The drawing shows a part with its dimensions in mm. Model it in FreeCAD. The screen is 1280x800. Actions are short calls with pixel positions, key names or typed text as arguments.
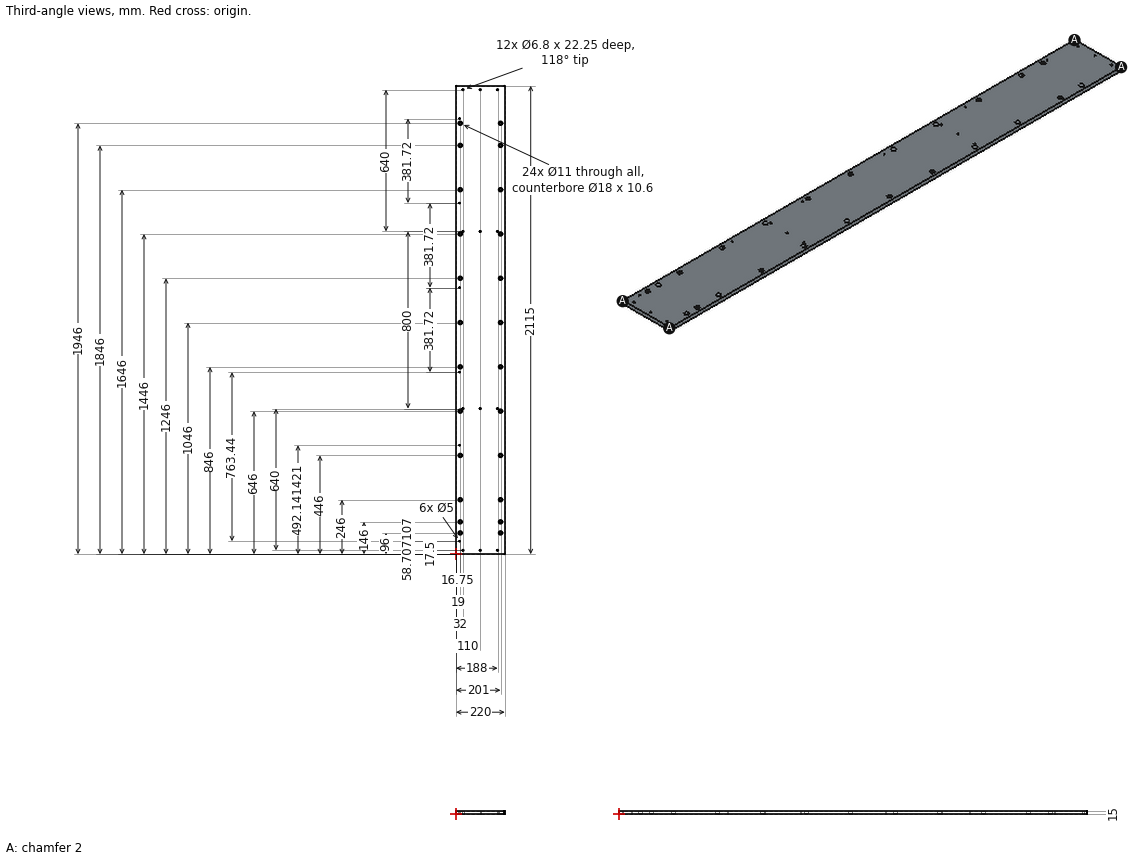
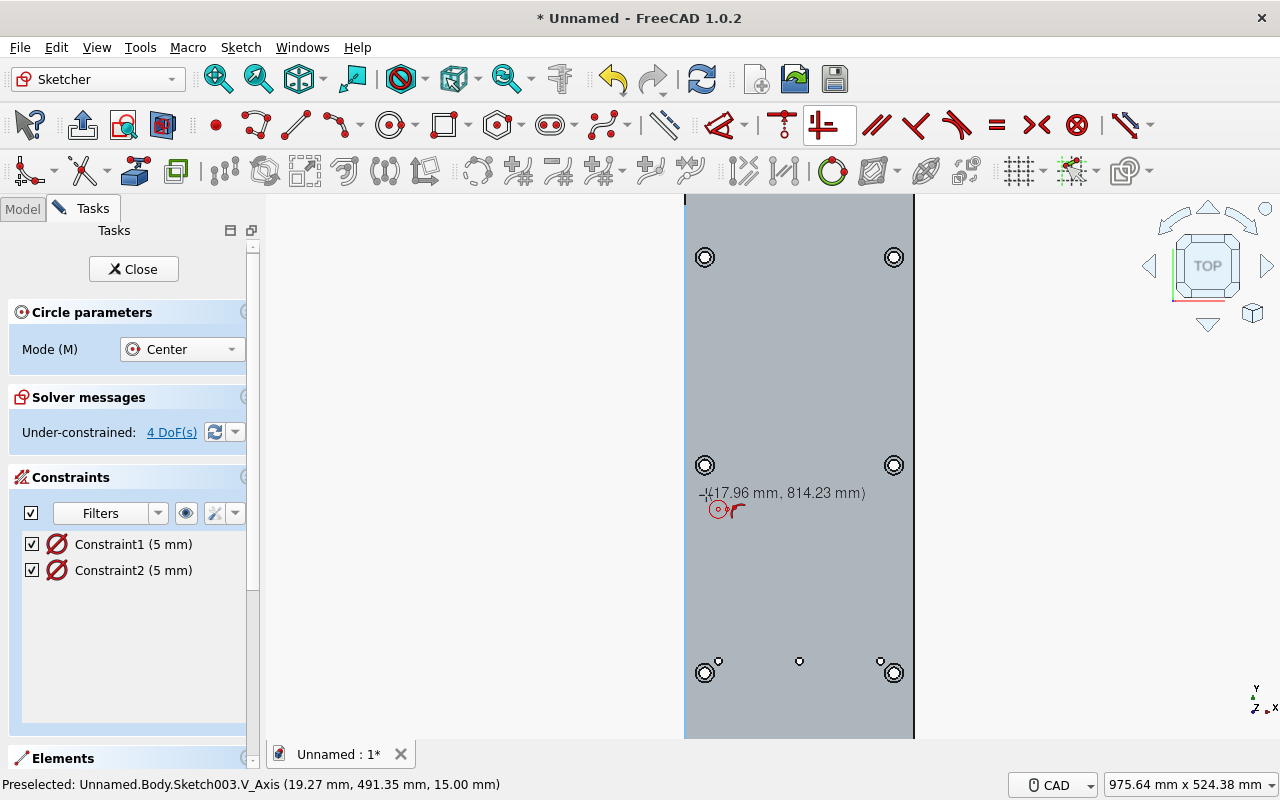
click(703, 490)
move(704, 488)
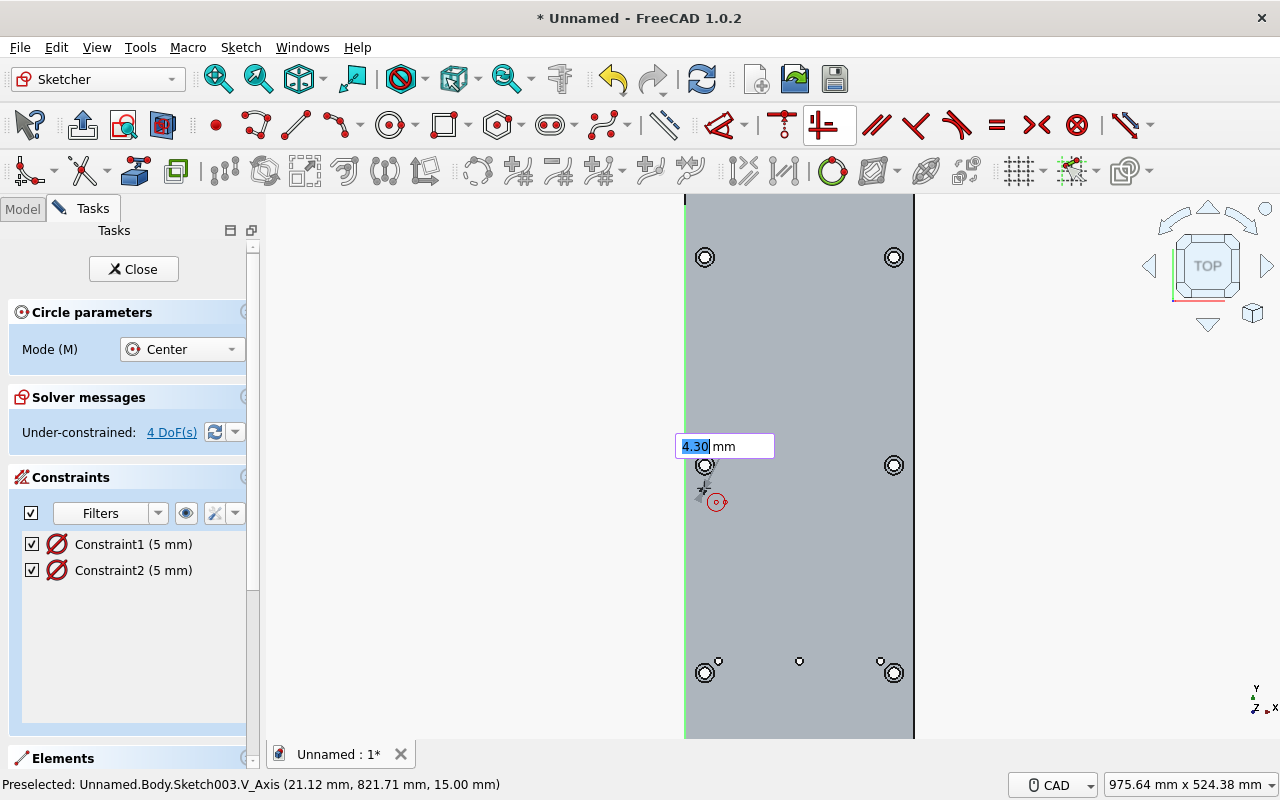
text(5)
key(Return)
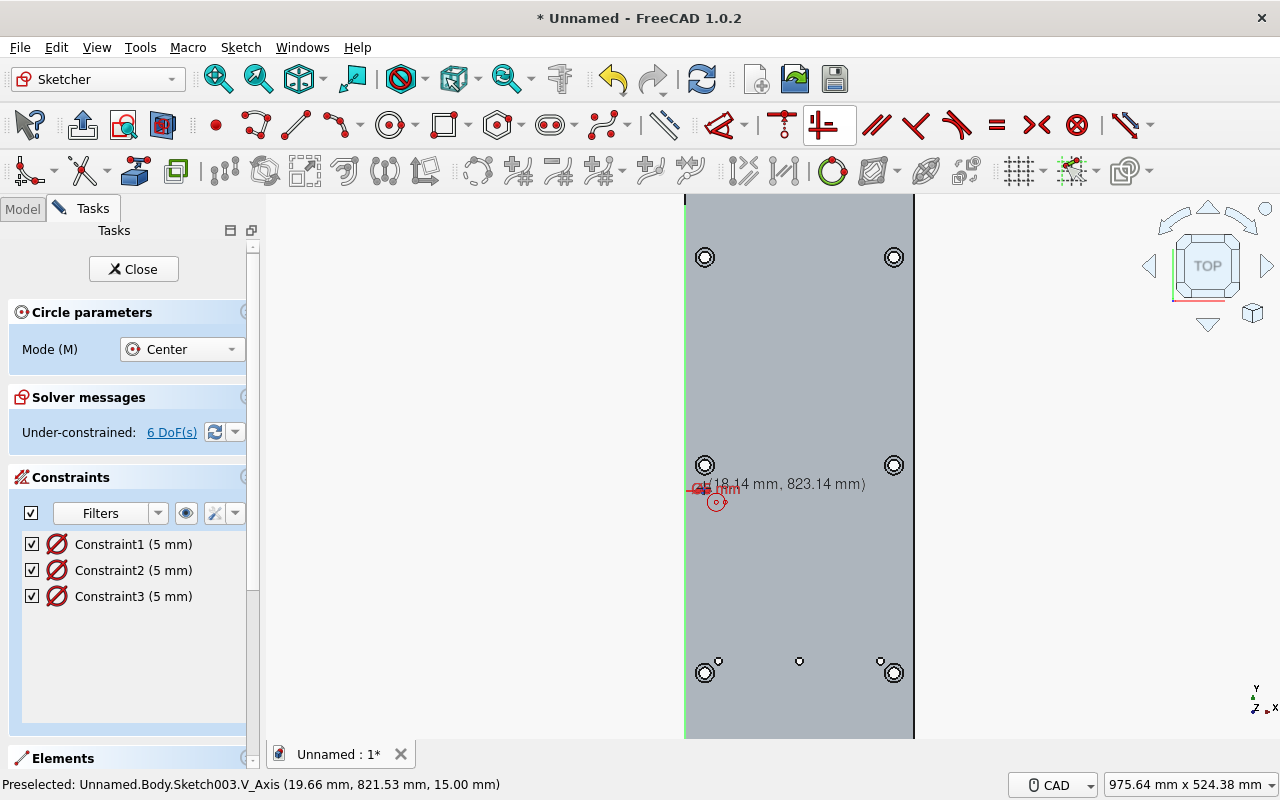
scroll(706, 495, down, 9)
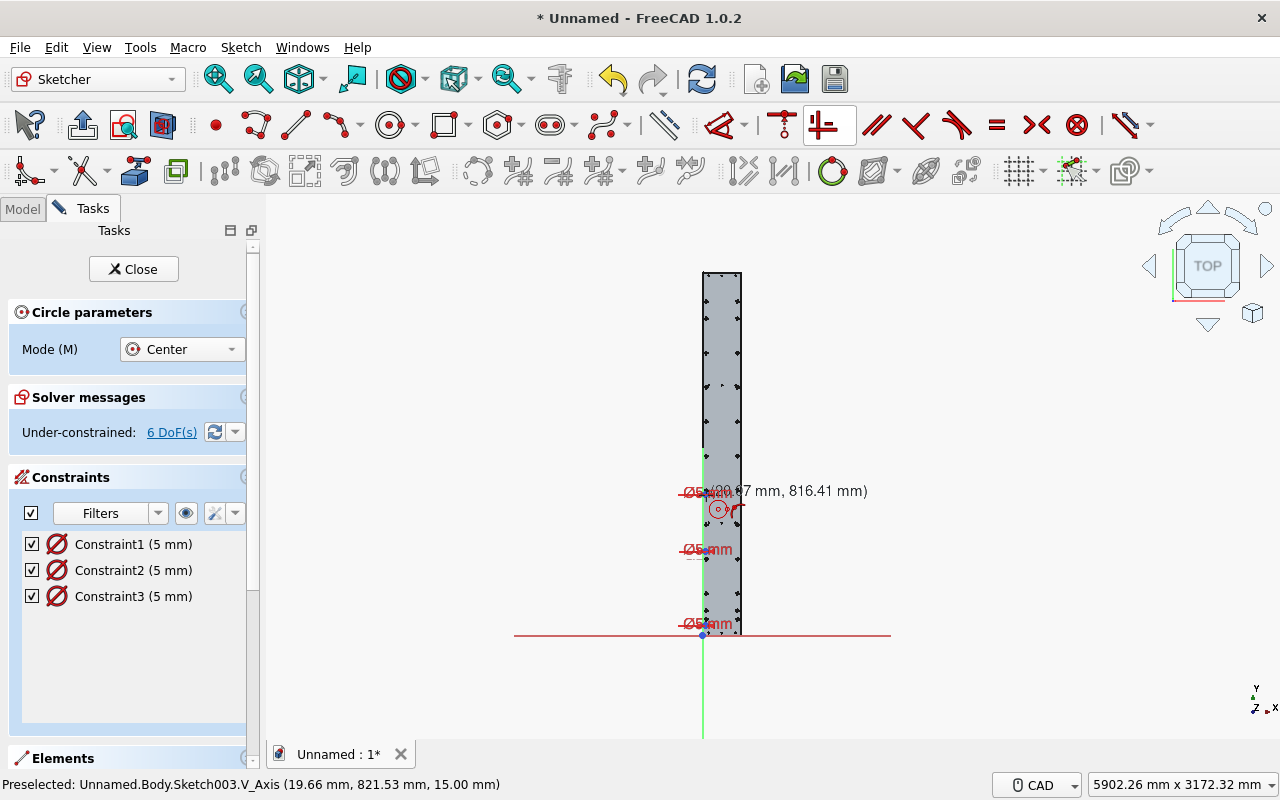
scroll(706, 429, up, 20)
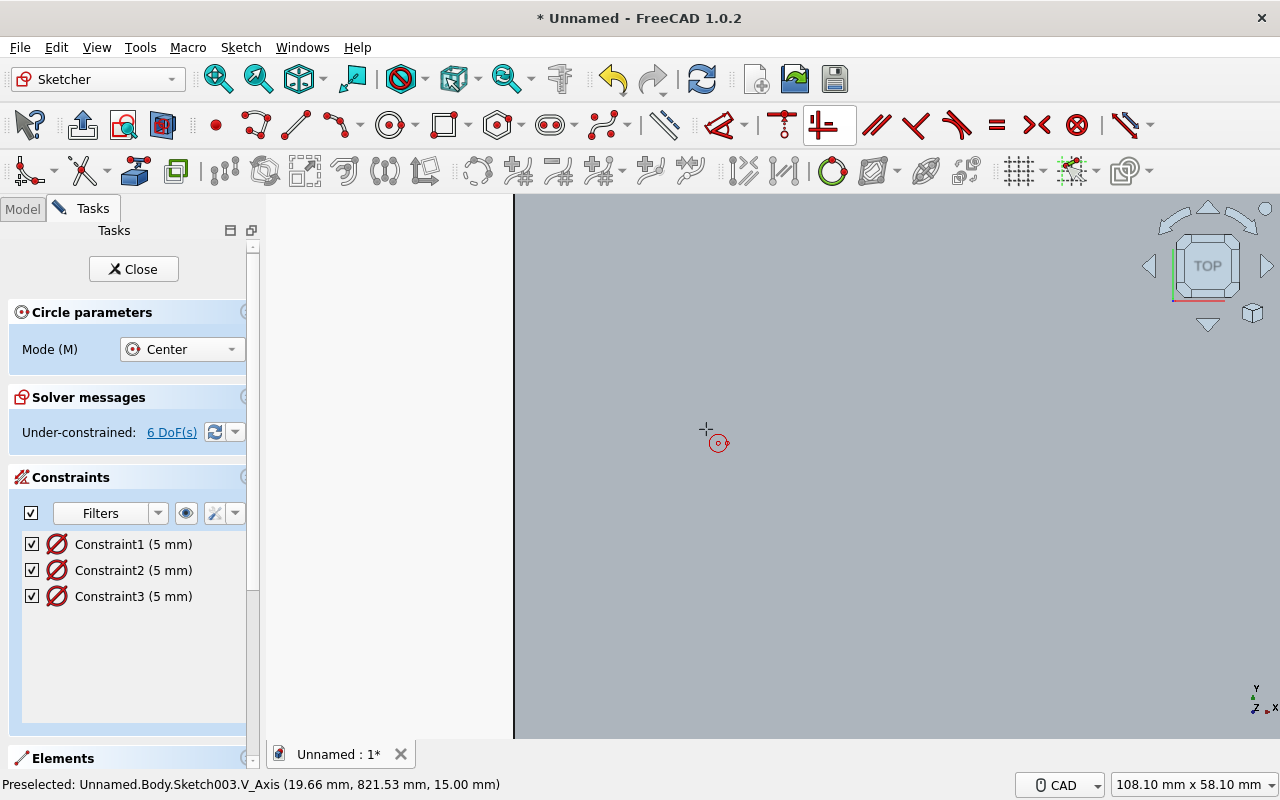
scroll(704, 466, down, 15)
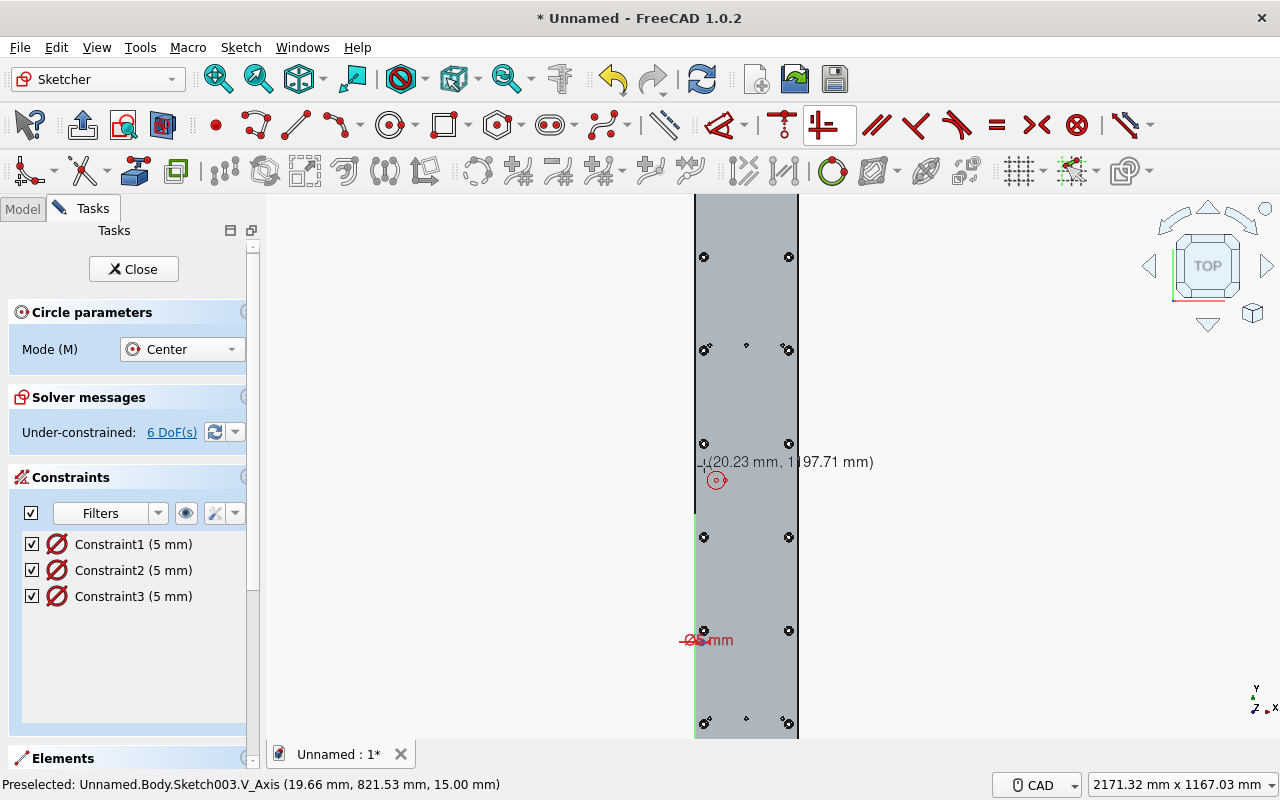
scroll(707, 409, down, 5)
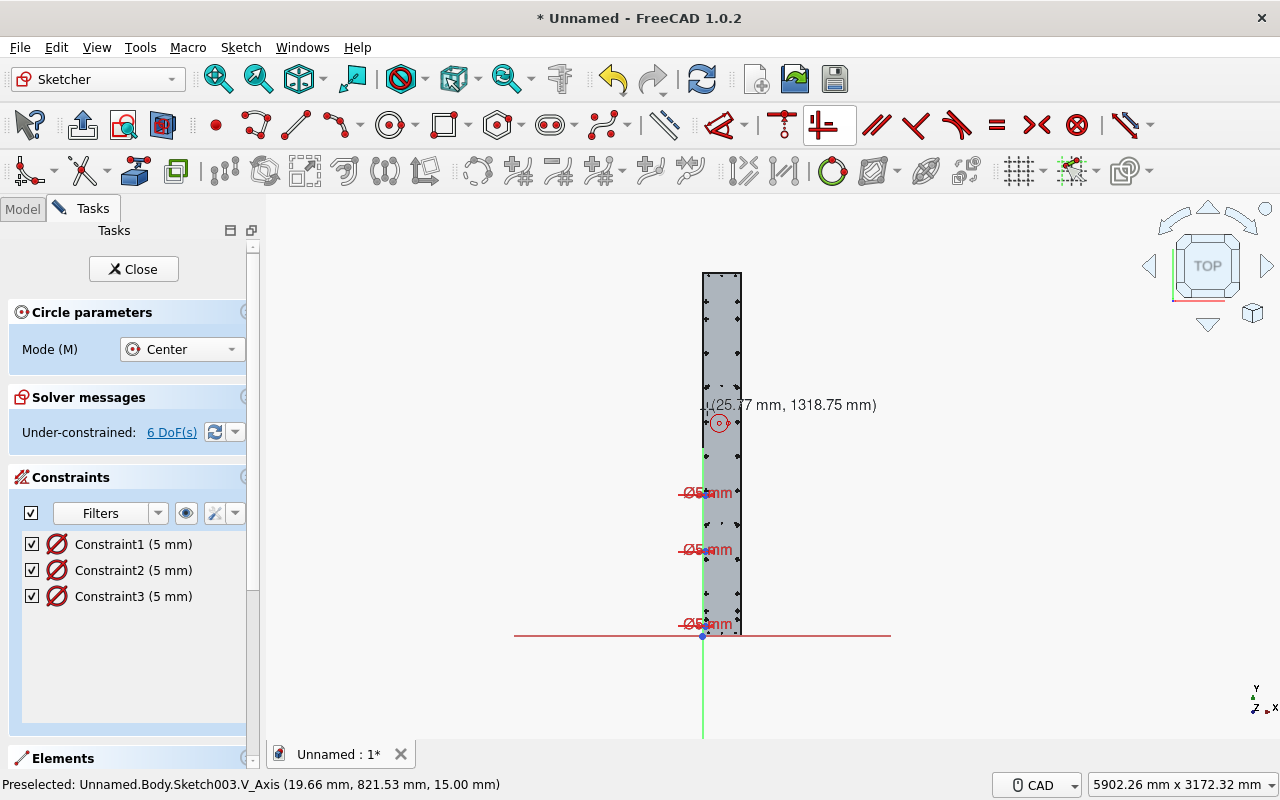
scroll(706, 429, up, 9)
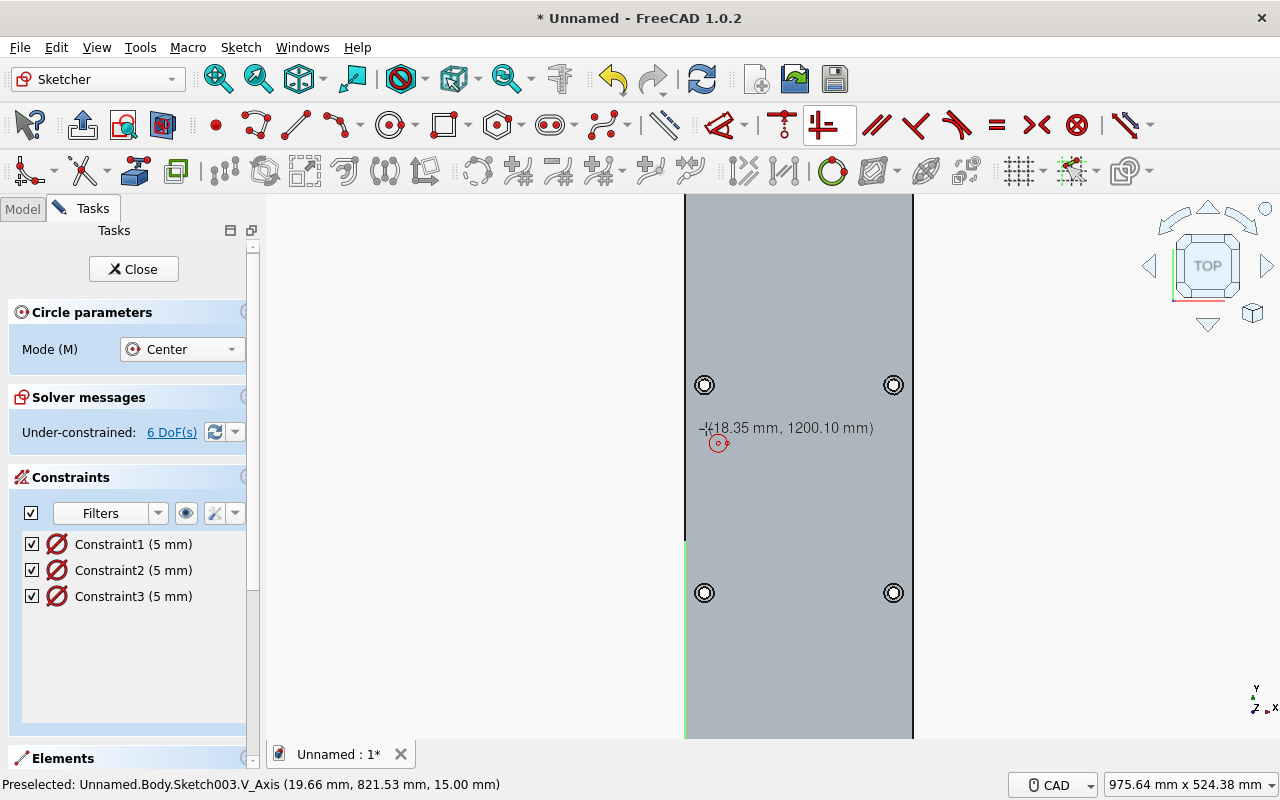
click(702, 429)
move(704, 427)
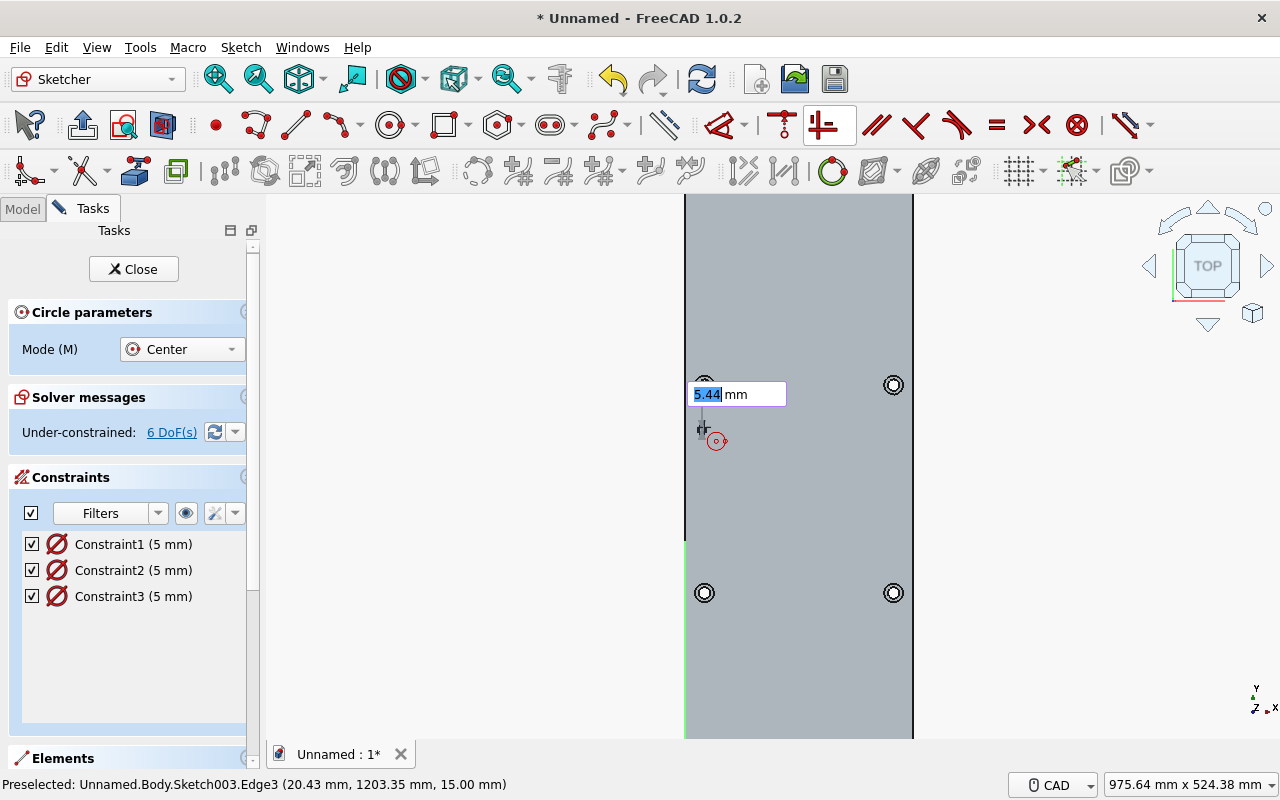
text(5)
key(Return)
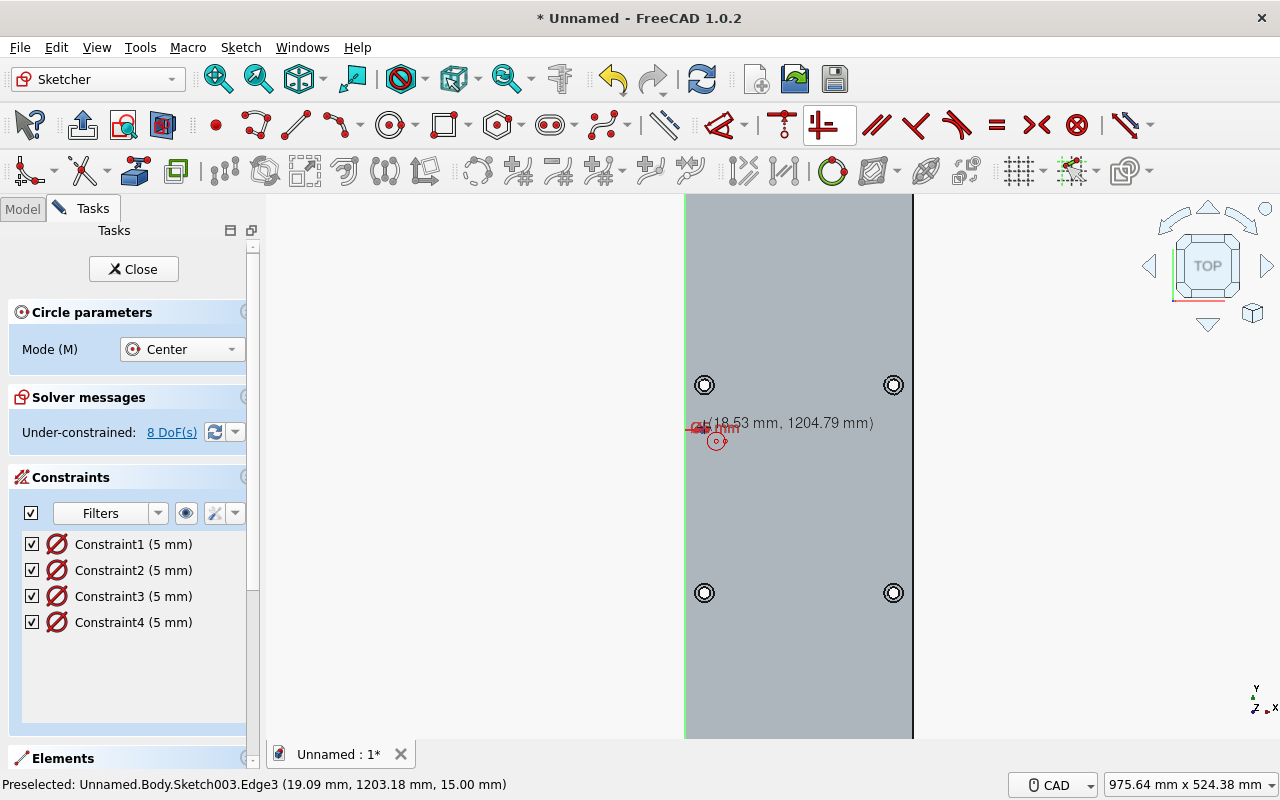
scroll(706, 429, down, 9)